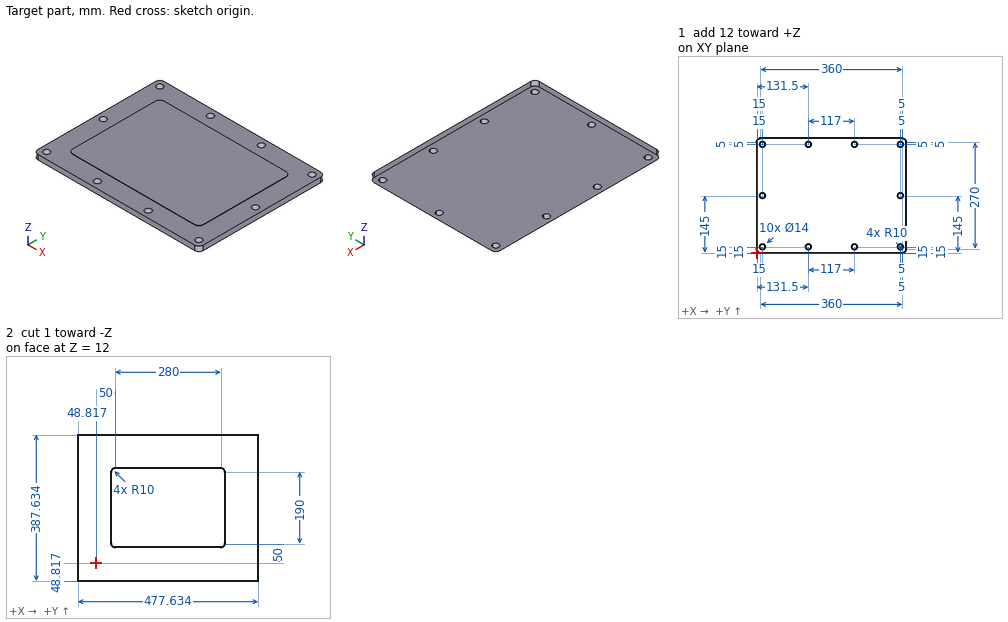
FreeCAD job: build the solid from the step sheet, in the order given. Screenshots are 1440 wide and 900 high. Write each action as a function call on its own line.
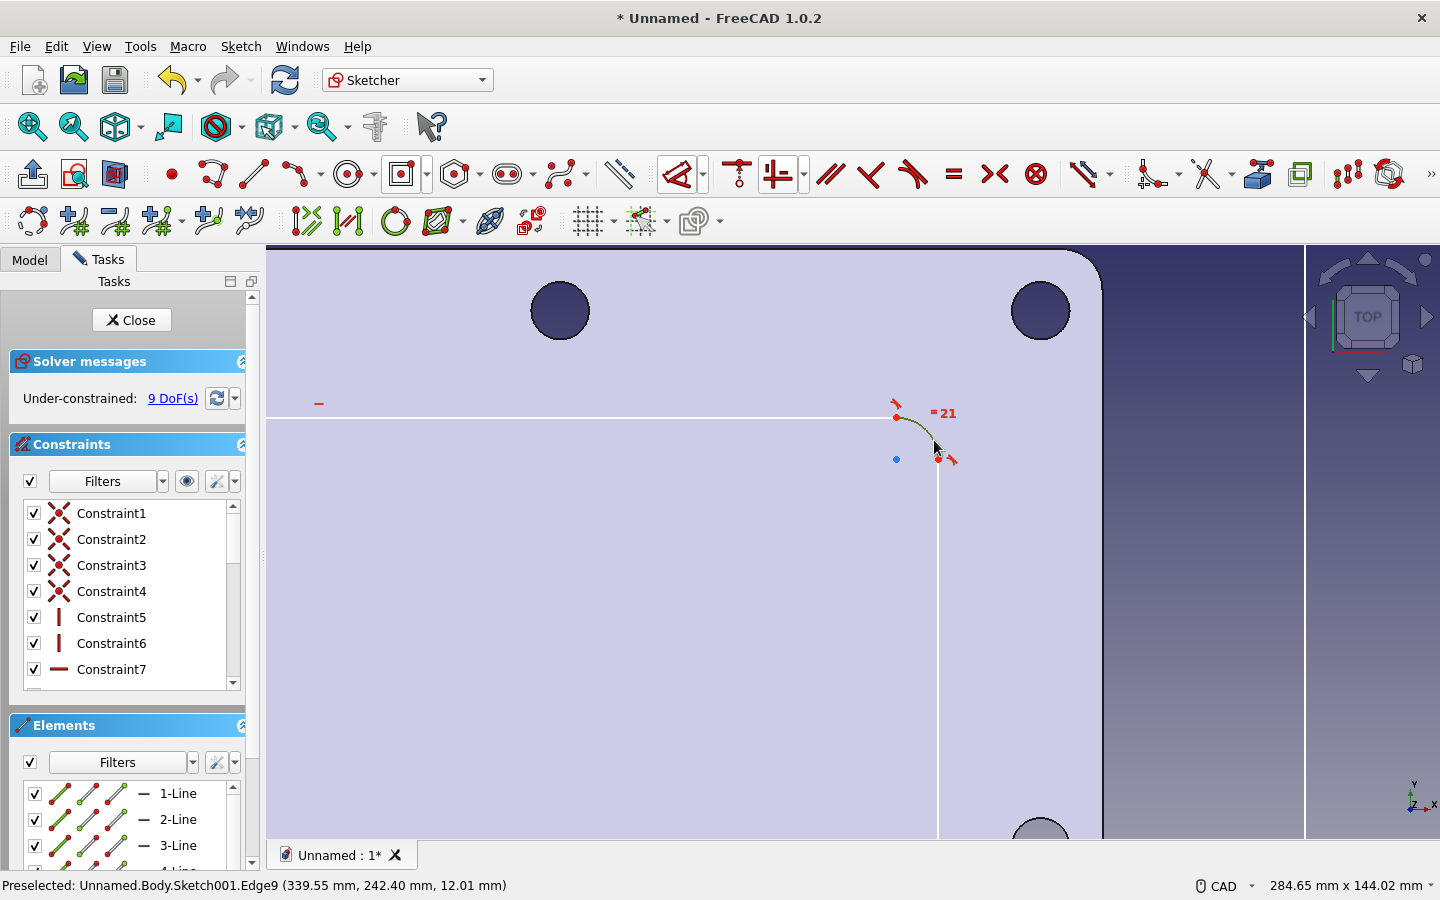
key(k)
key(r)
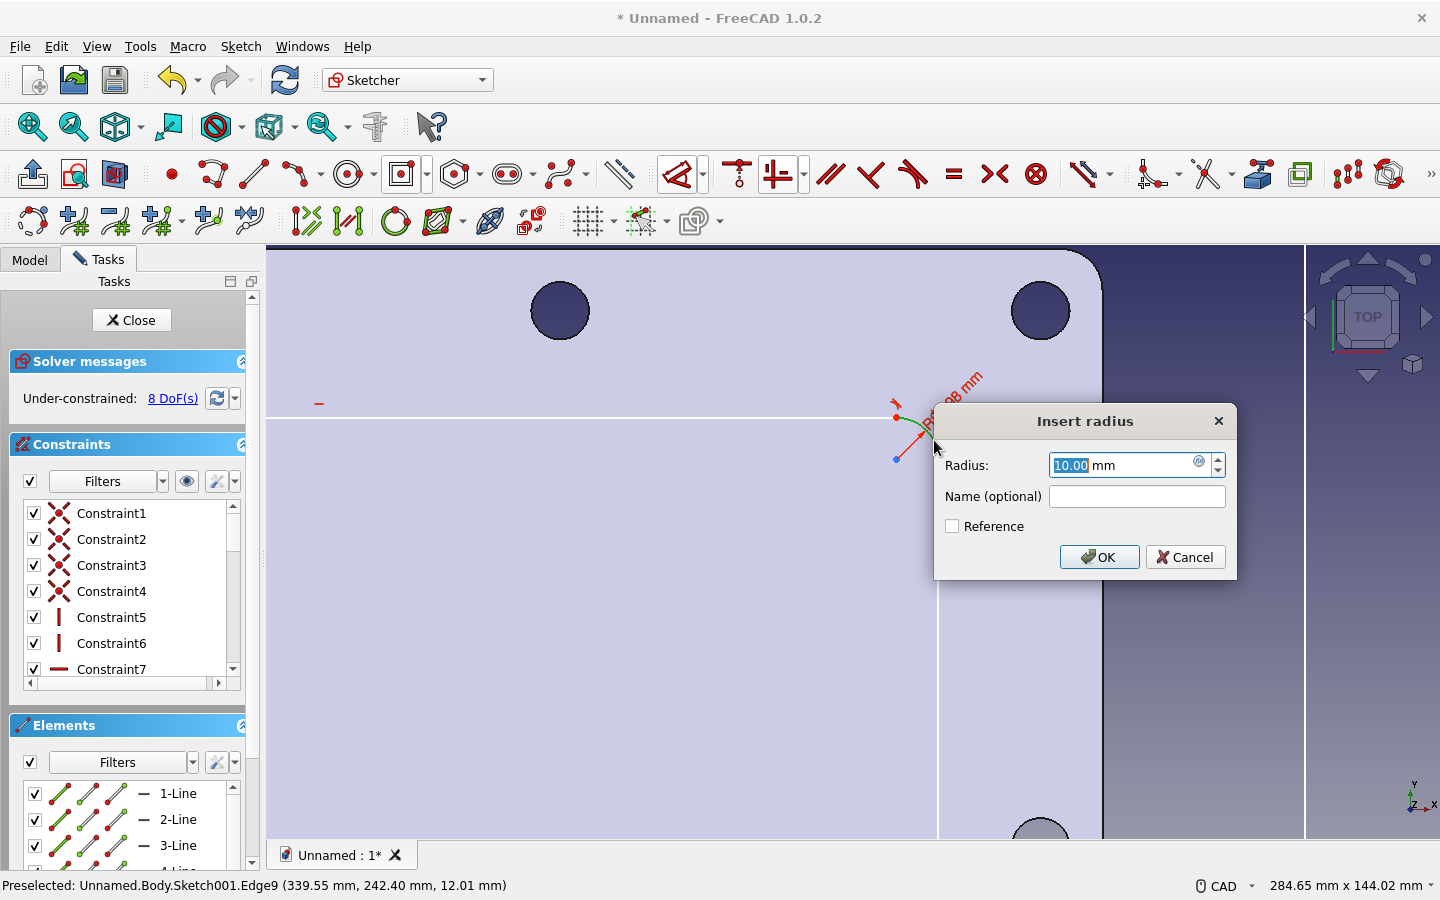
text(10)
key(Return)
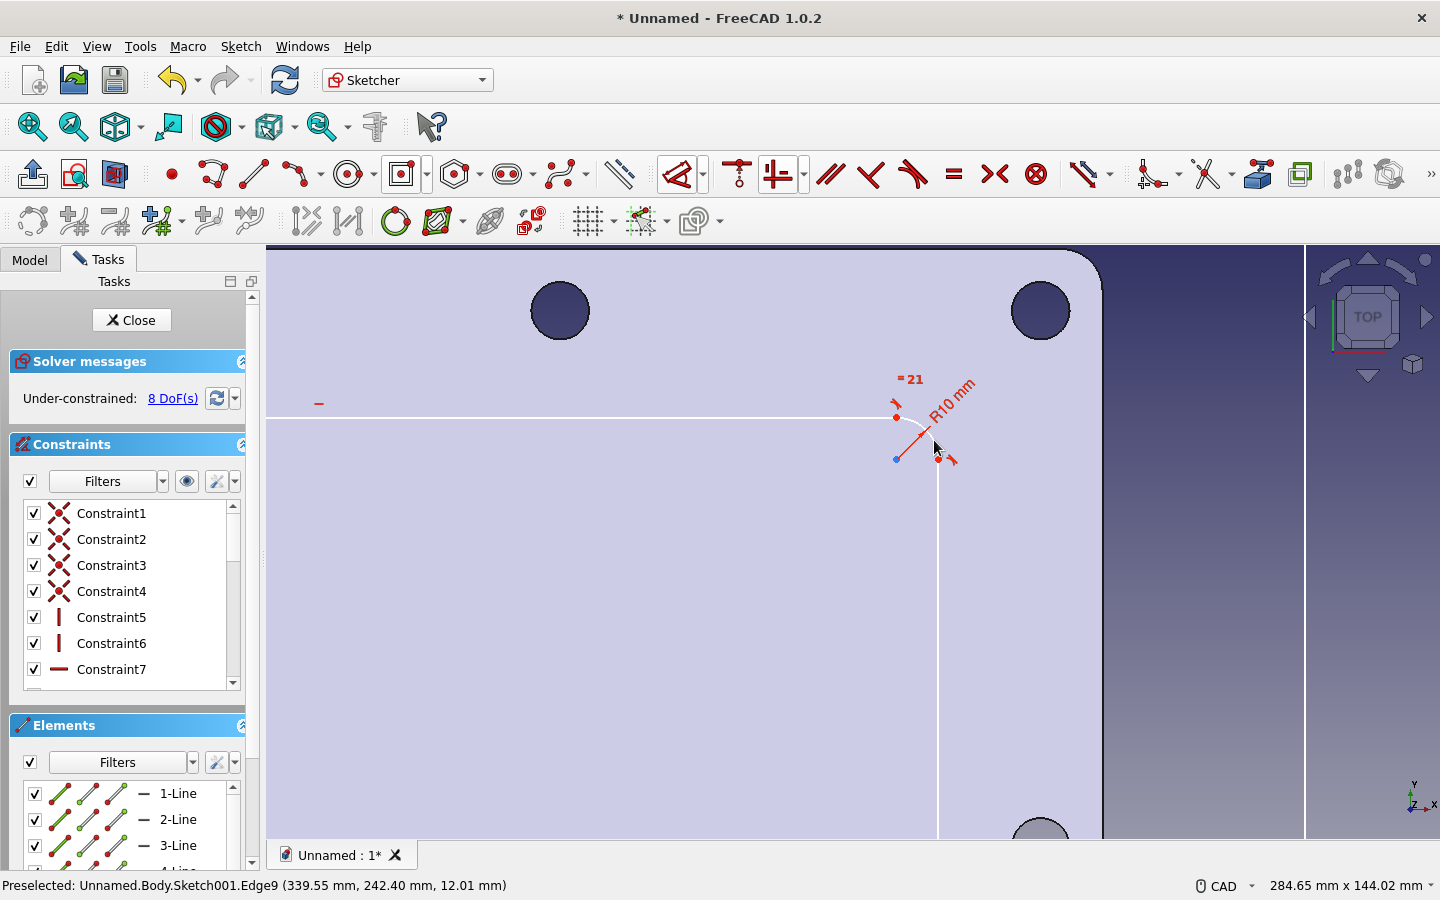
click(550, 418)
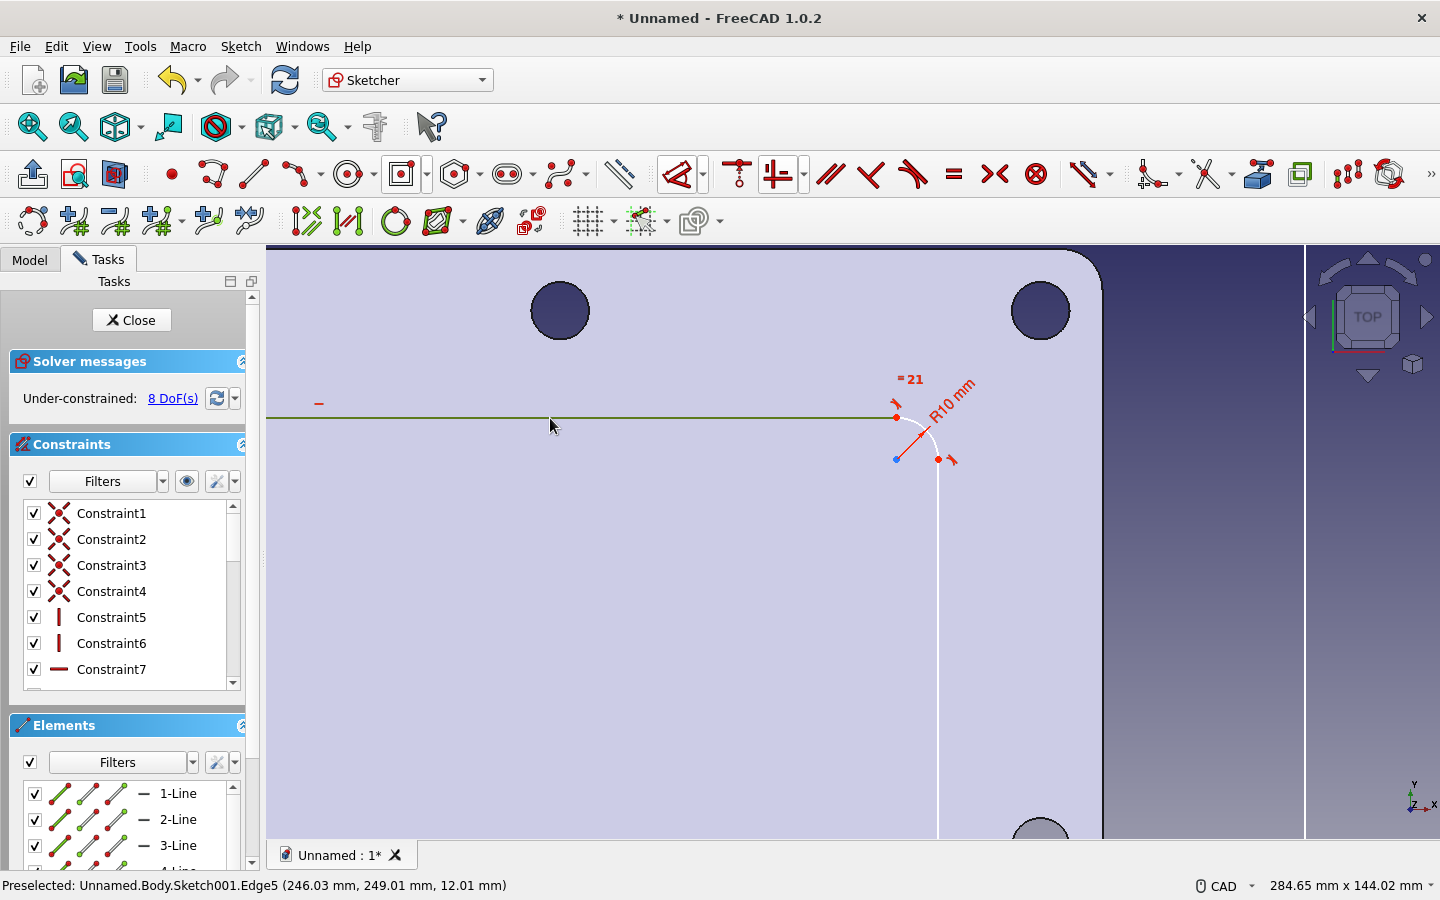
click(702, 174)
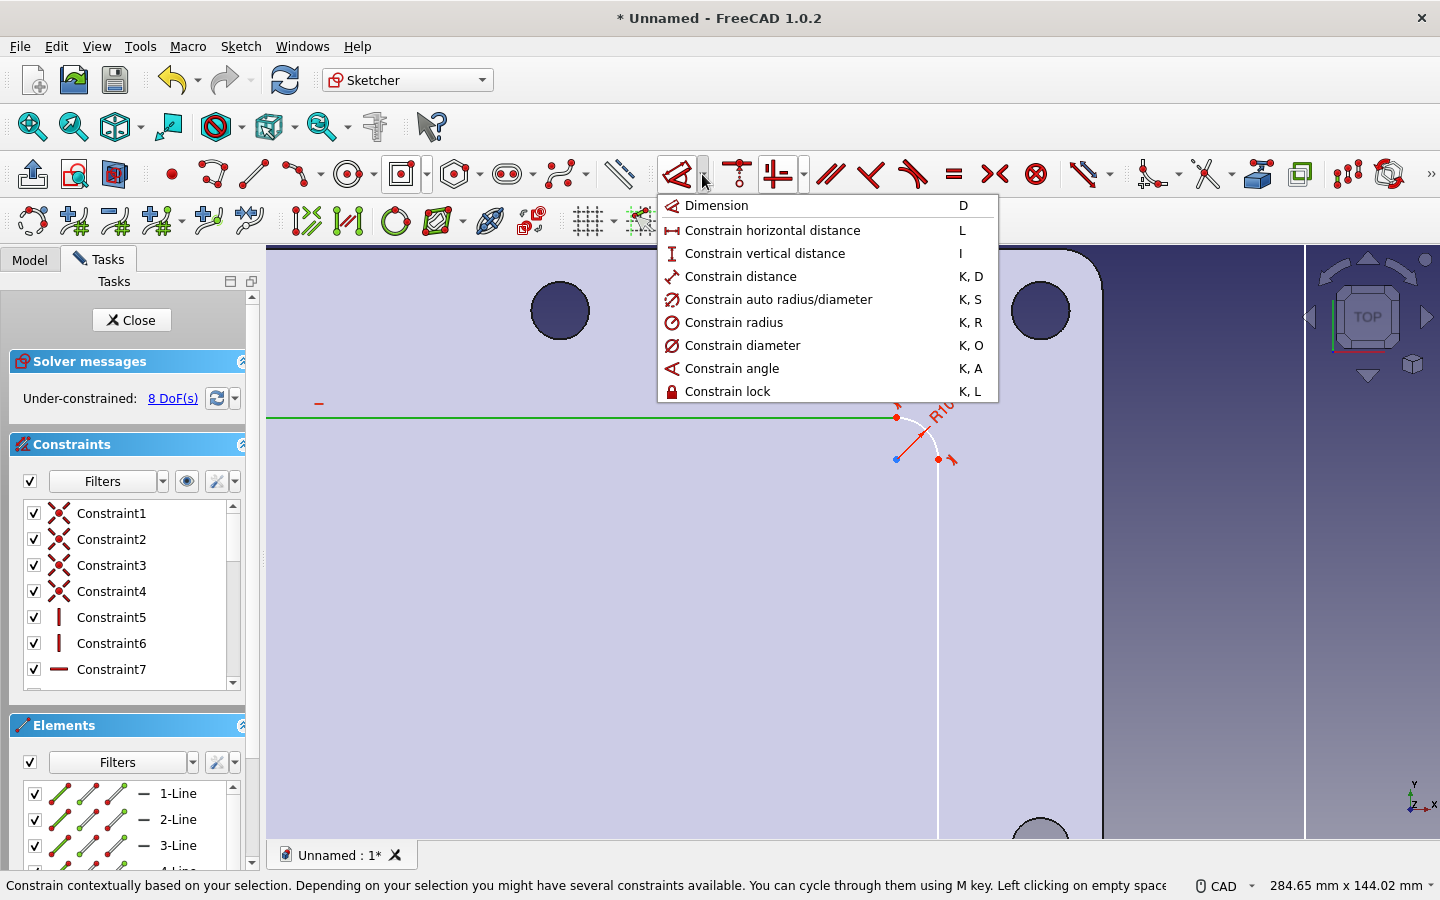
click(828, 230)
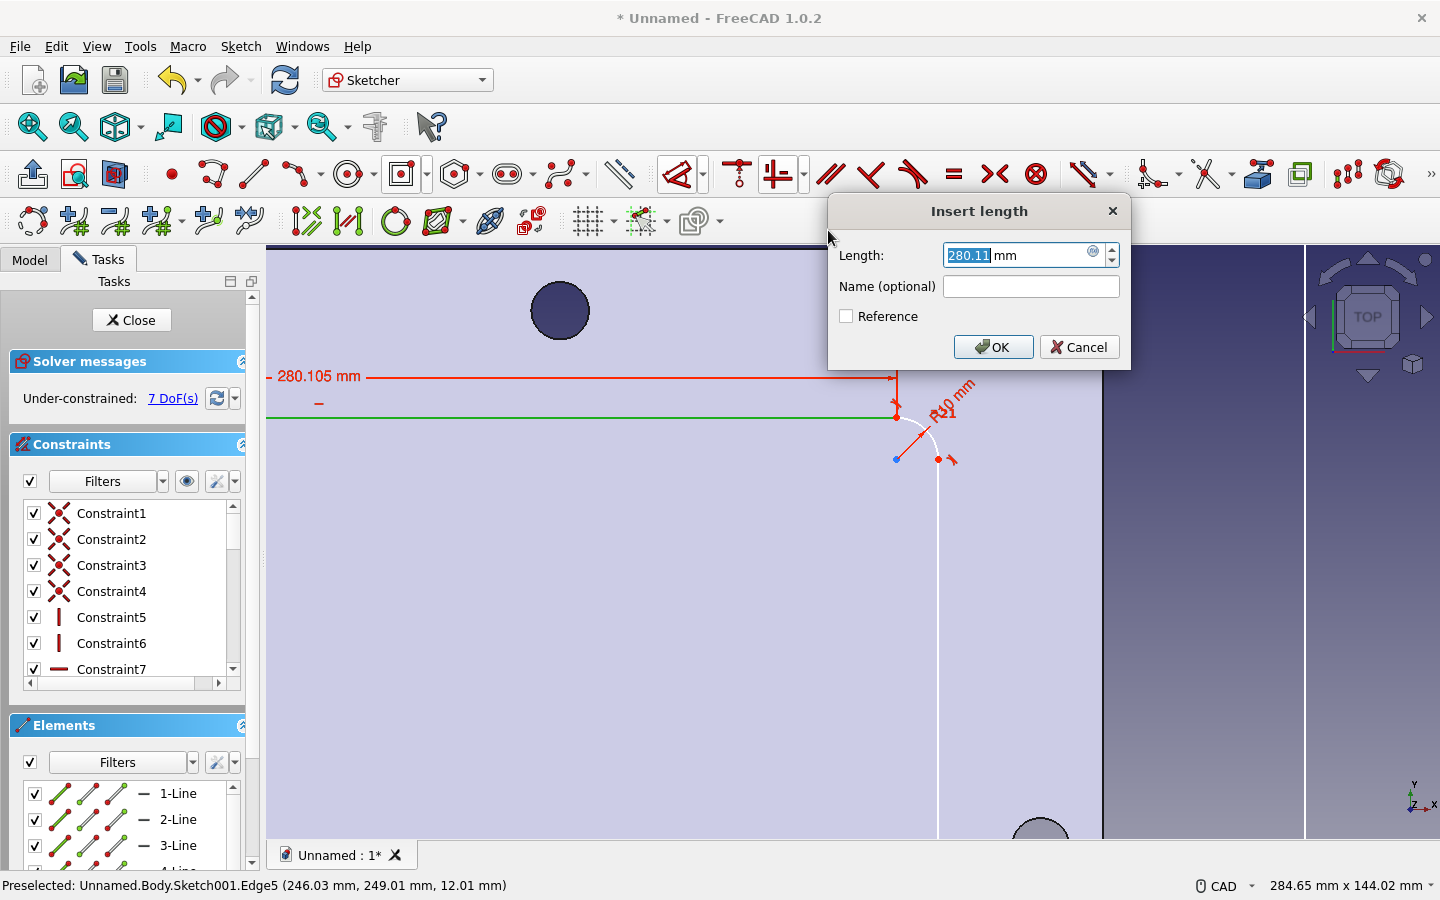
text(280)
key(Return)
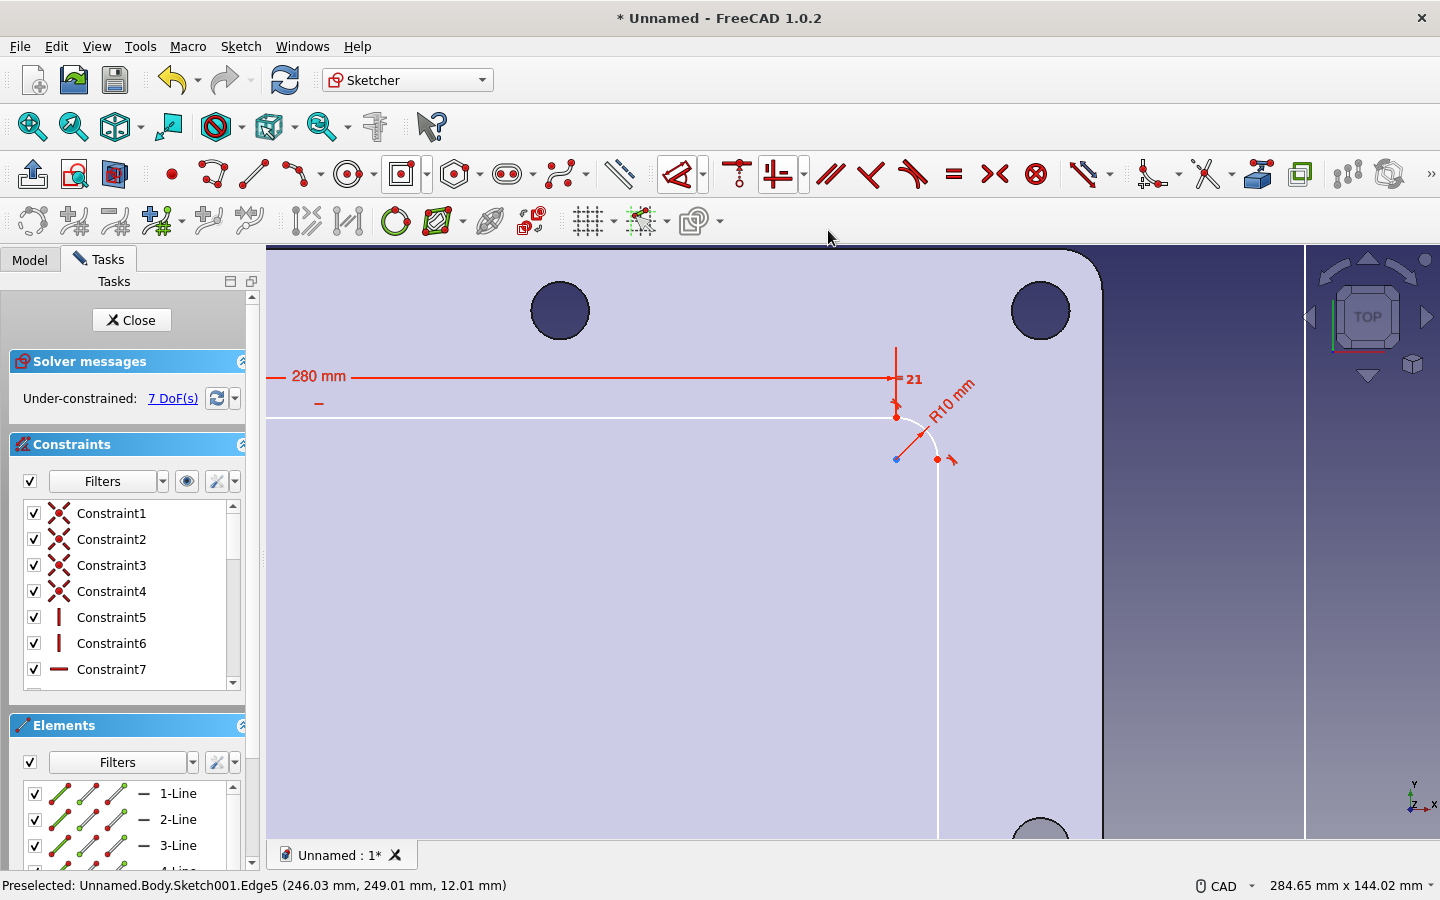
click(938, 694)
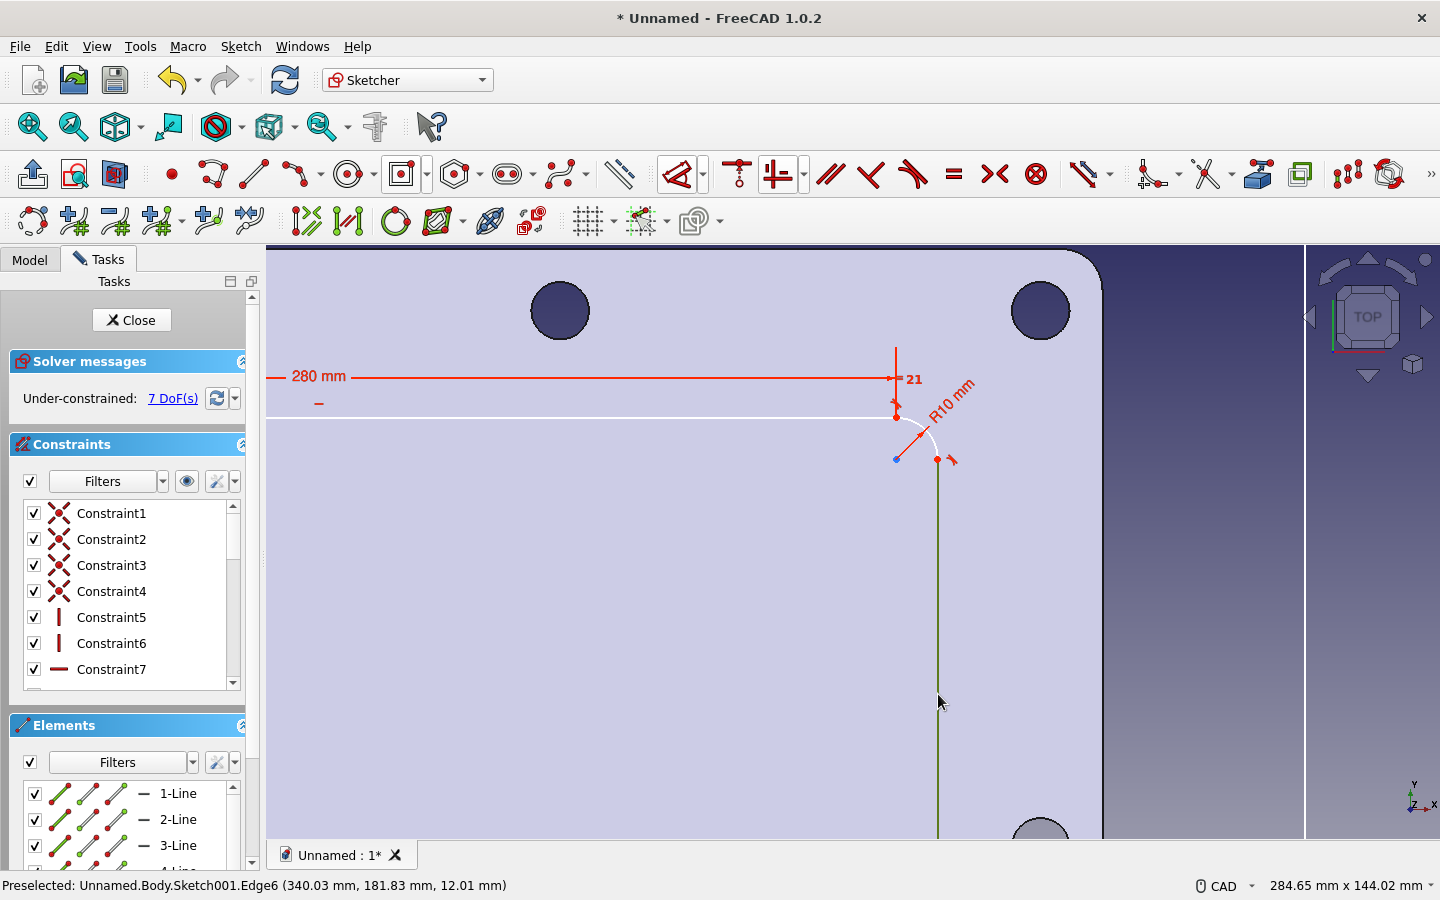
click(702, 174)